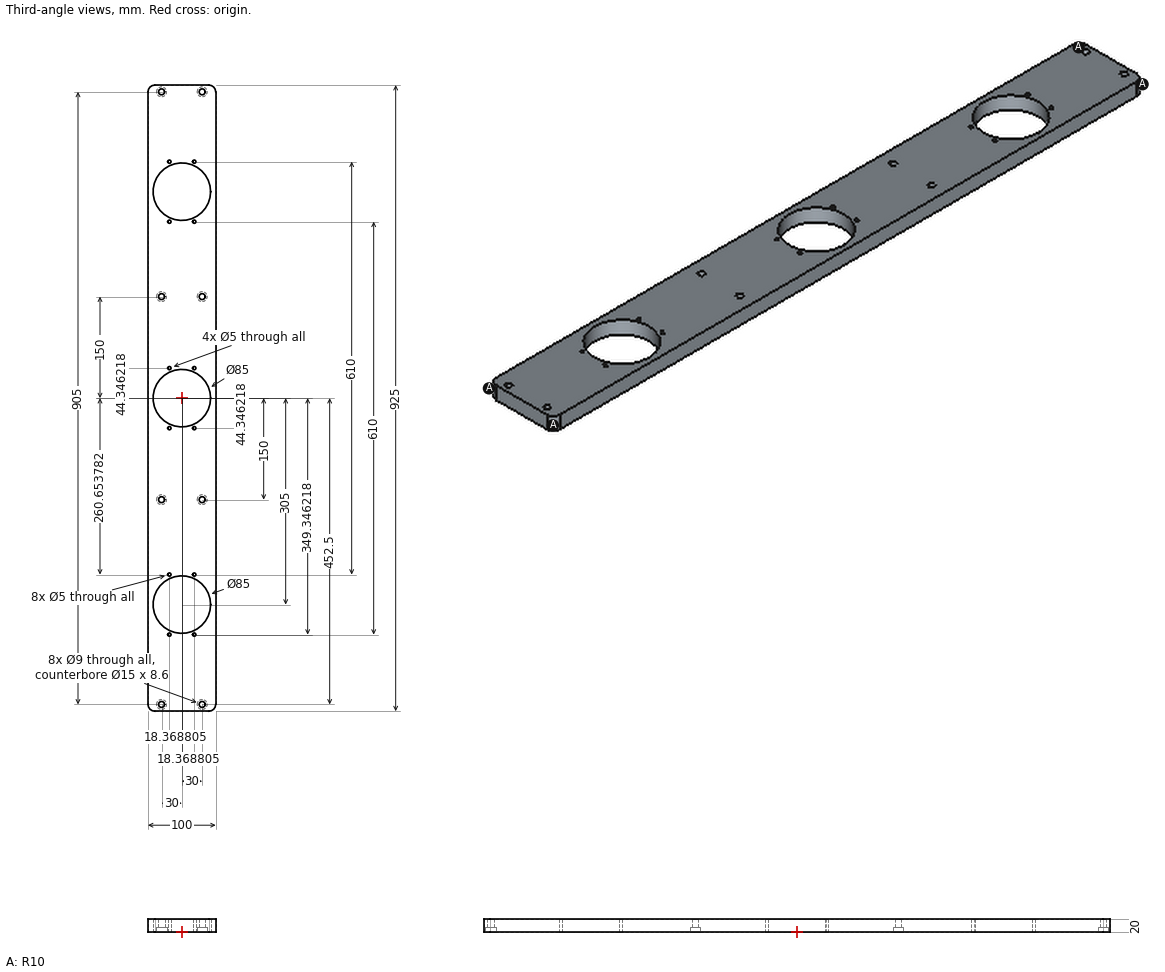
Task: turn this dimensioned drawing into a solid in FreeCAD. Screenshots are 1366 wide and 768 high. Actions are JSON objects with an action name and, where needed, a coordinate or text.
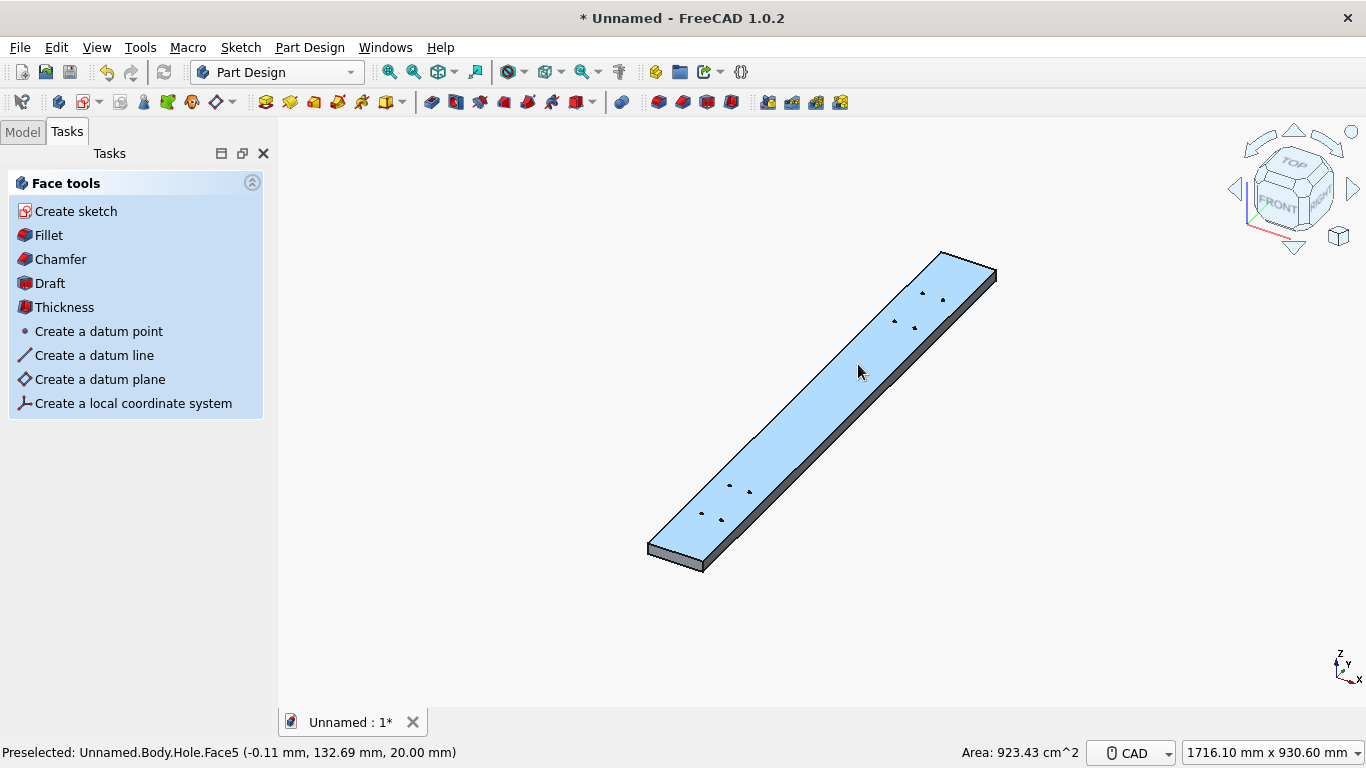
{"action": "left_click", "coordinate": [84, 102]}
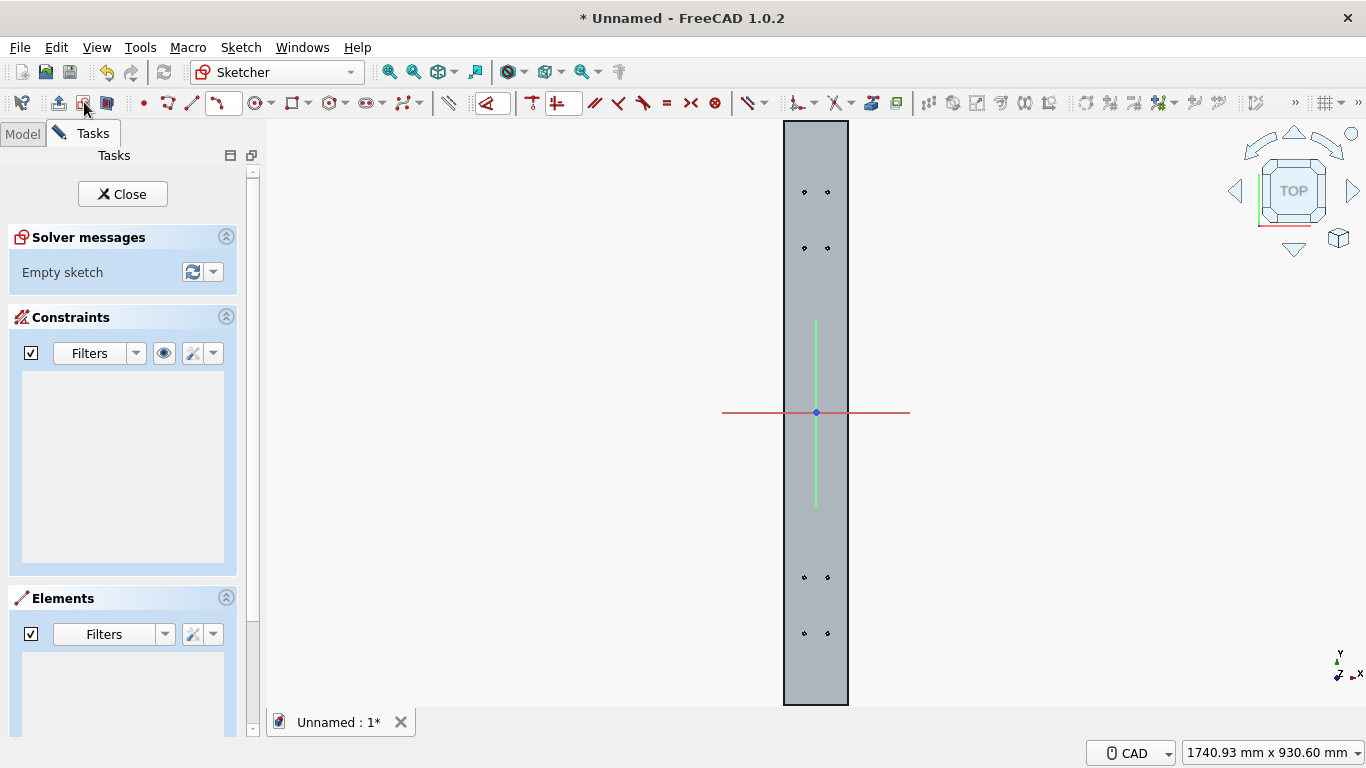
{"action": "scroll", "coordinate": [827, 636], "scroll_direction": "up", "scroll_amount": 10}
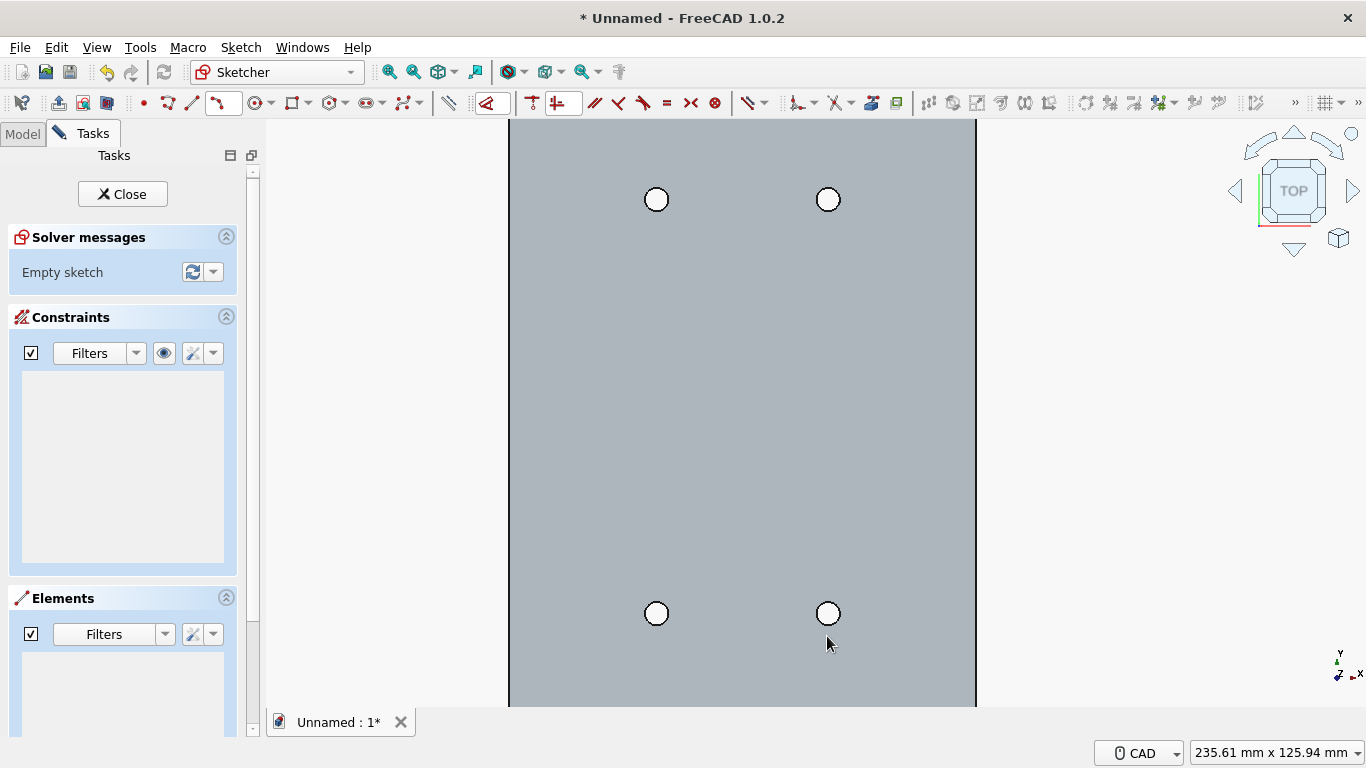
{"action": "left_click", "coordinate": [256, 104]}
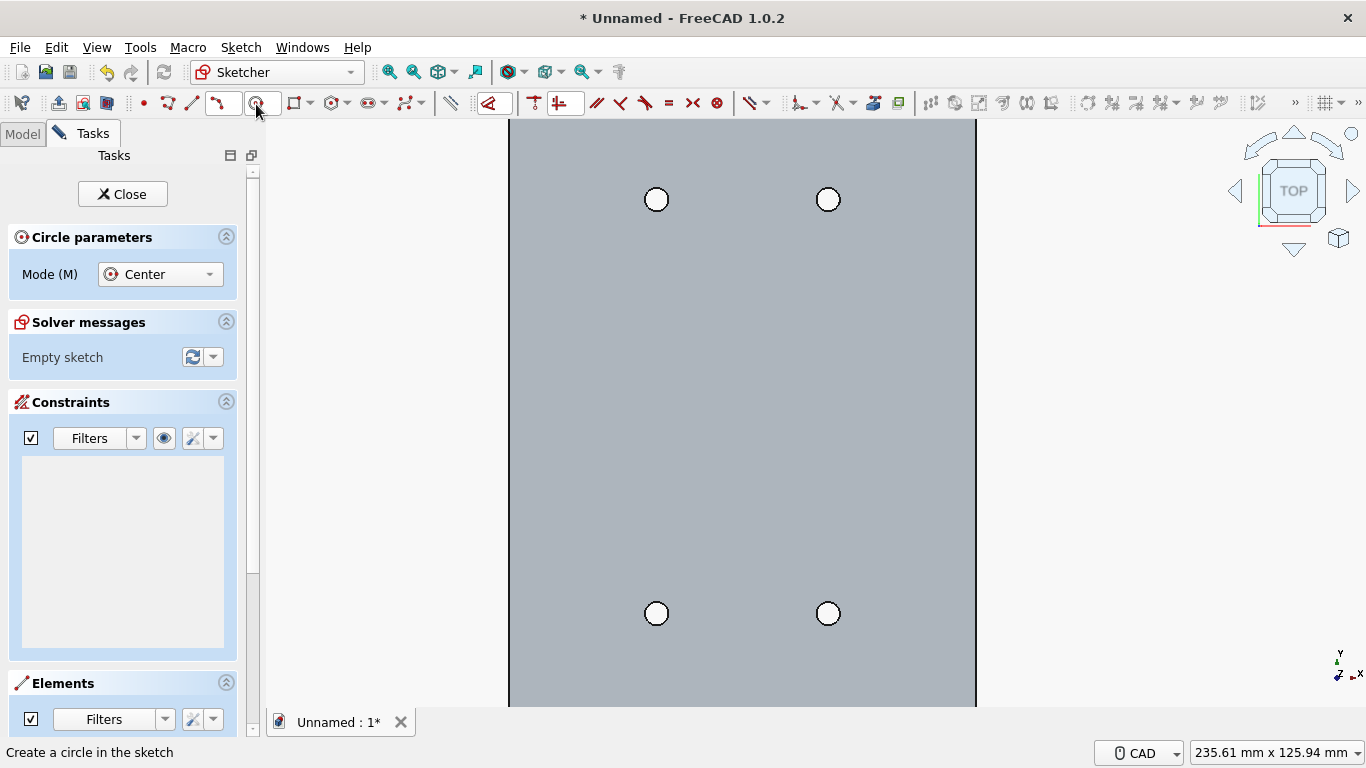
{"action": "left_click", "coordinate": [742, 407]}
{"action": "left_click", "coordinate": [883, 266]}
{"action": "key", "text": "Escape"}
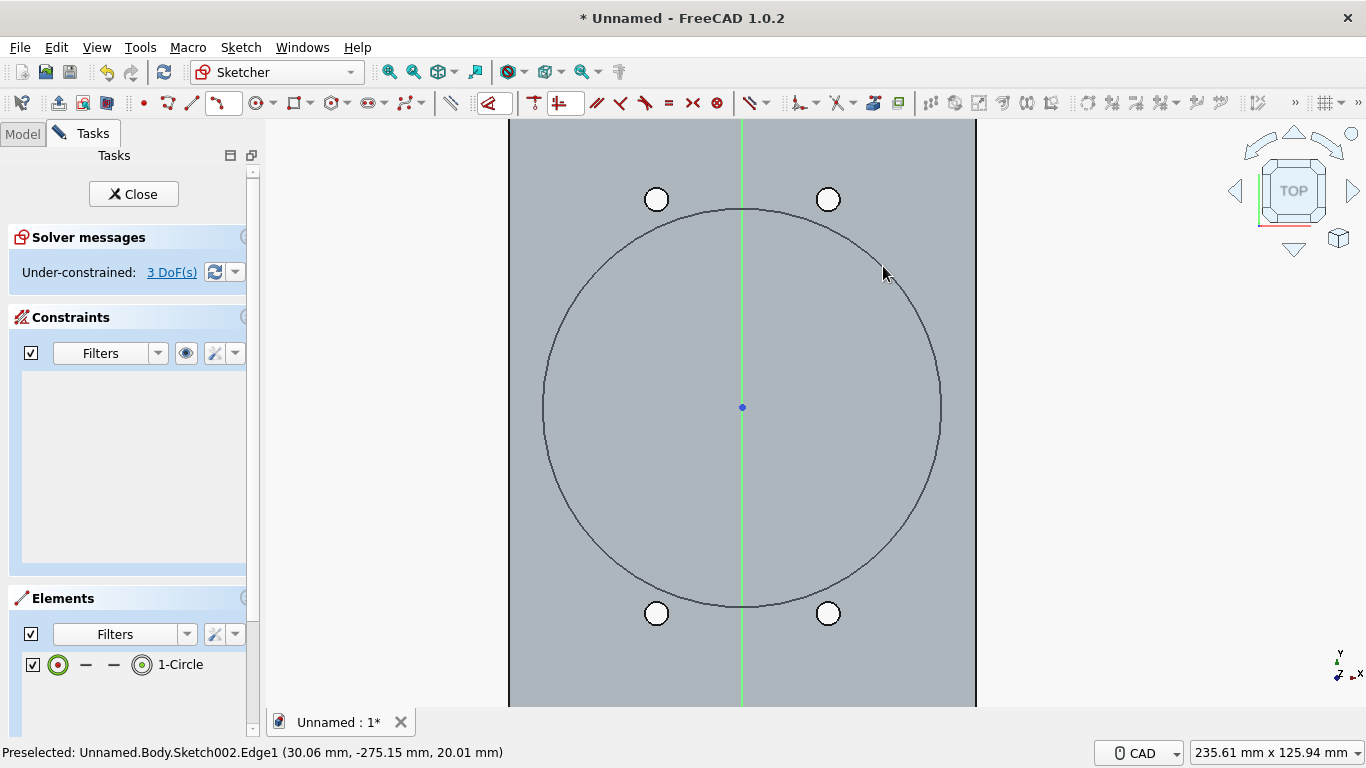
{"action": "left_click", "coordinate": [742, 408]}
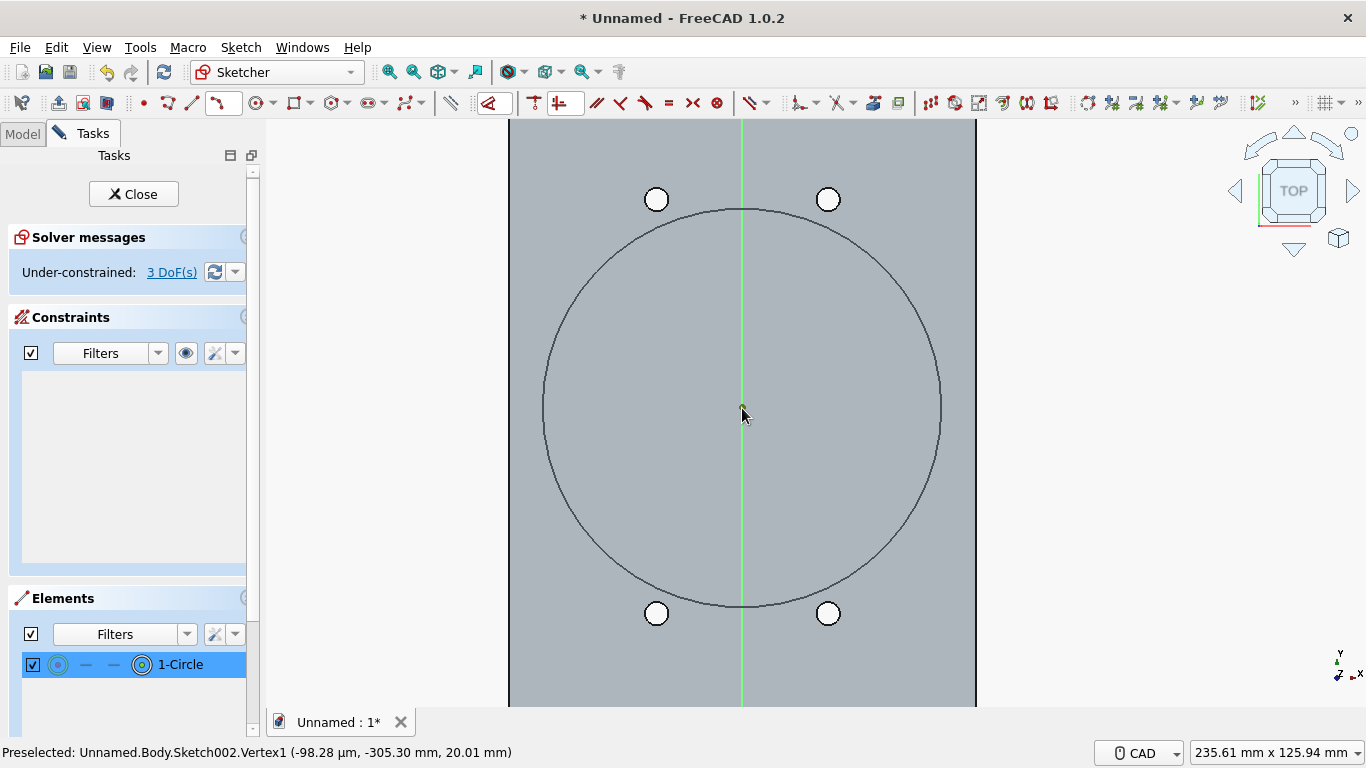
{"action": "left_click", "coordinate": [742, 641]}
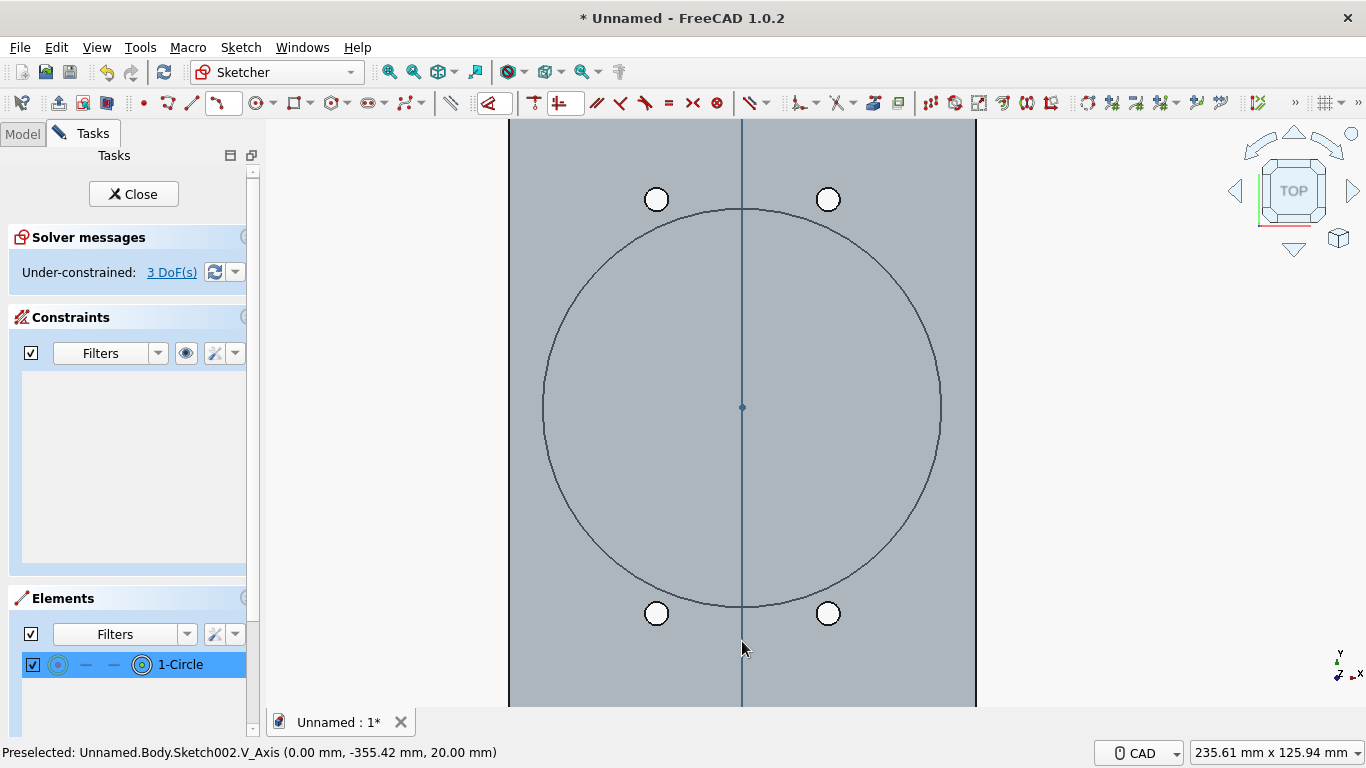
{"action": "key", "text": "c"}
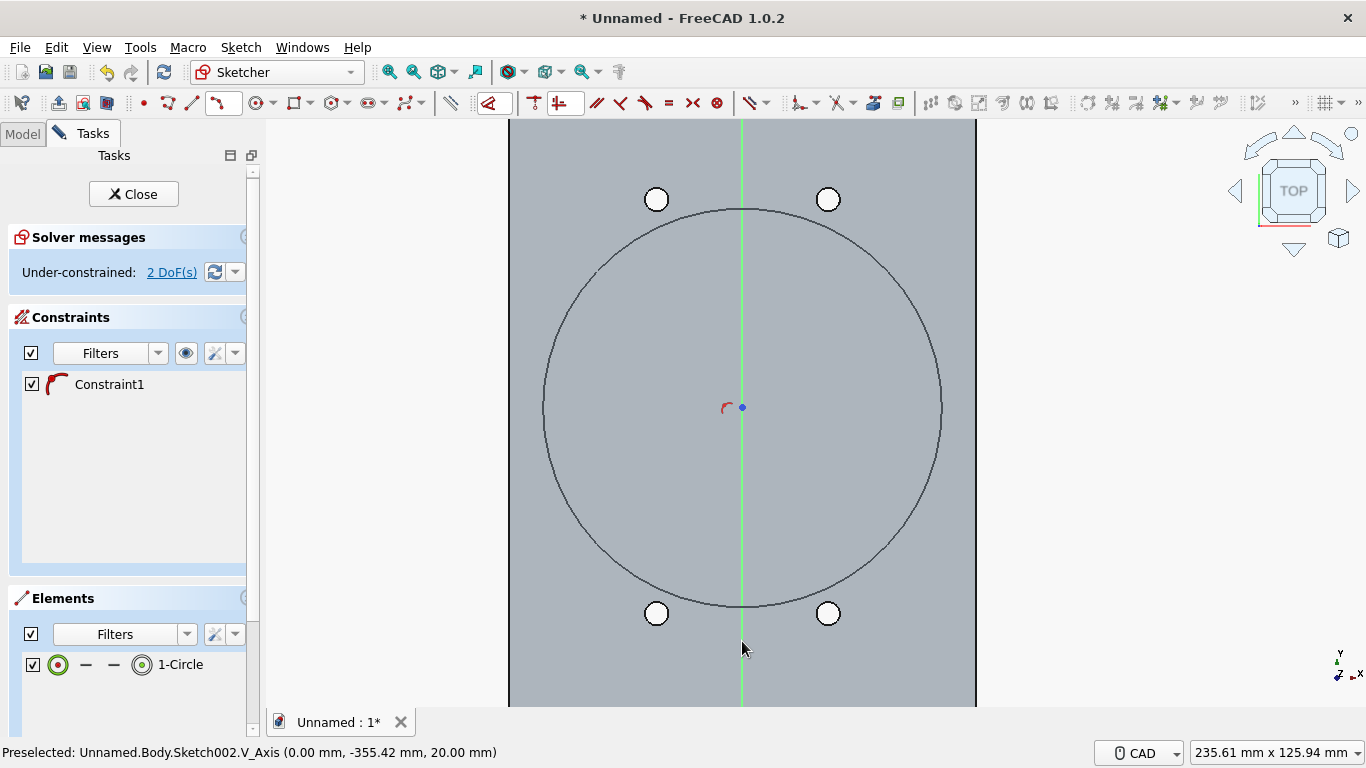
{"action": "key", "text": "d"}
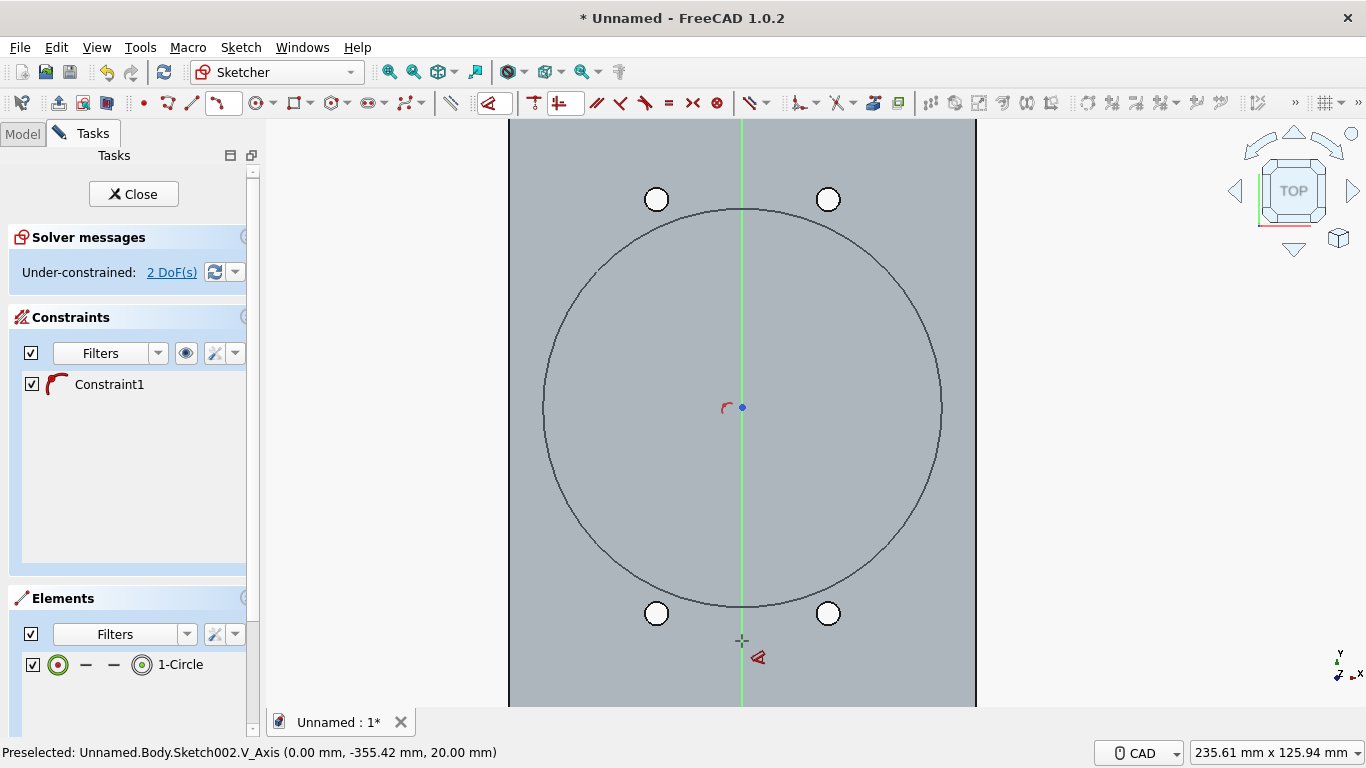
{"action": "left_click", "coordinate": [883, 267]}
{"action": "left_click", "coordinate": [906, 244]}